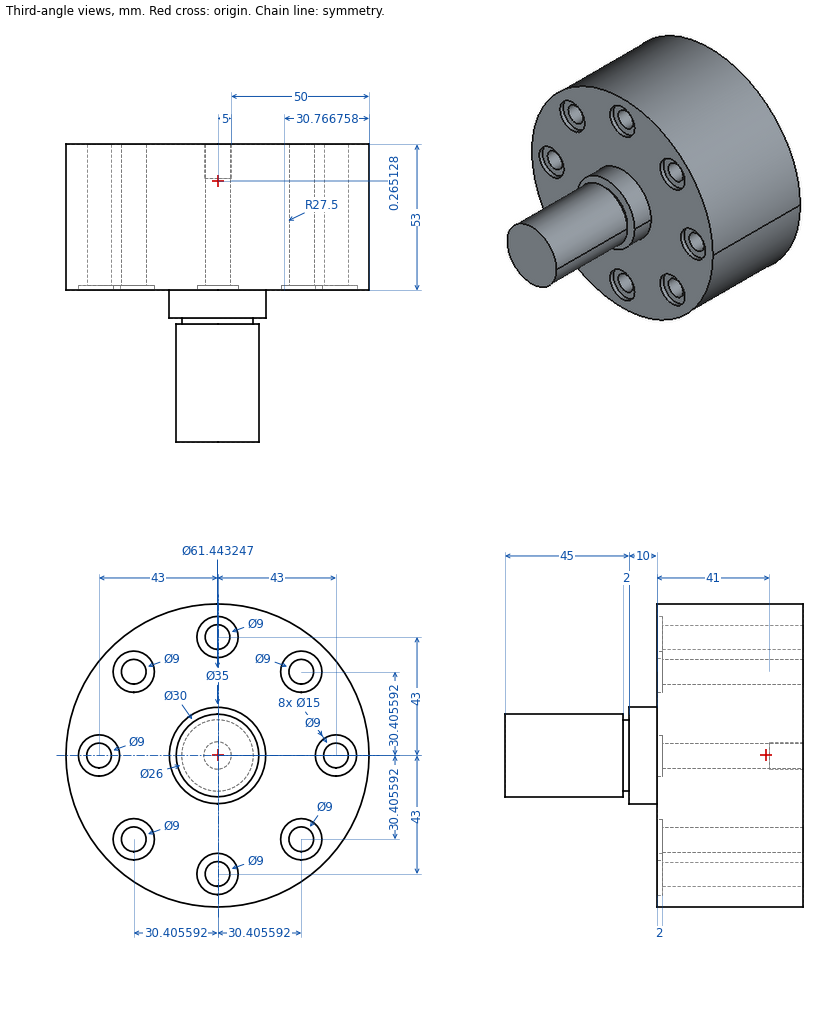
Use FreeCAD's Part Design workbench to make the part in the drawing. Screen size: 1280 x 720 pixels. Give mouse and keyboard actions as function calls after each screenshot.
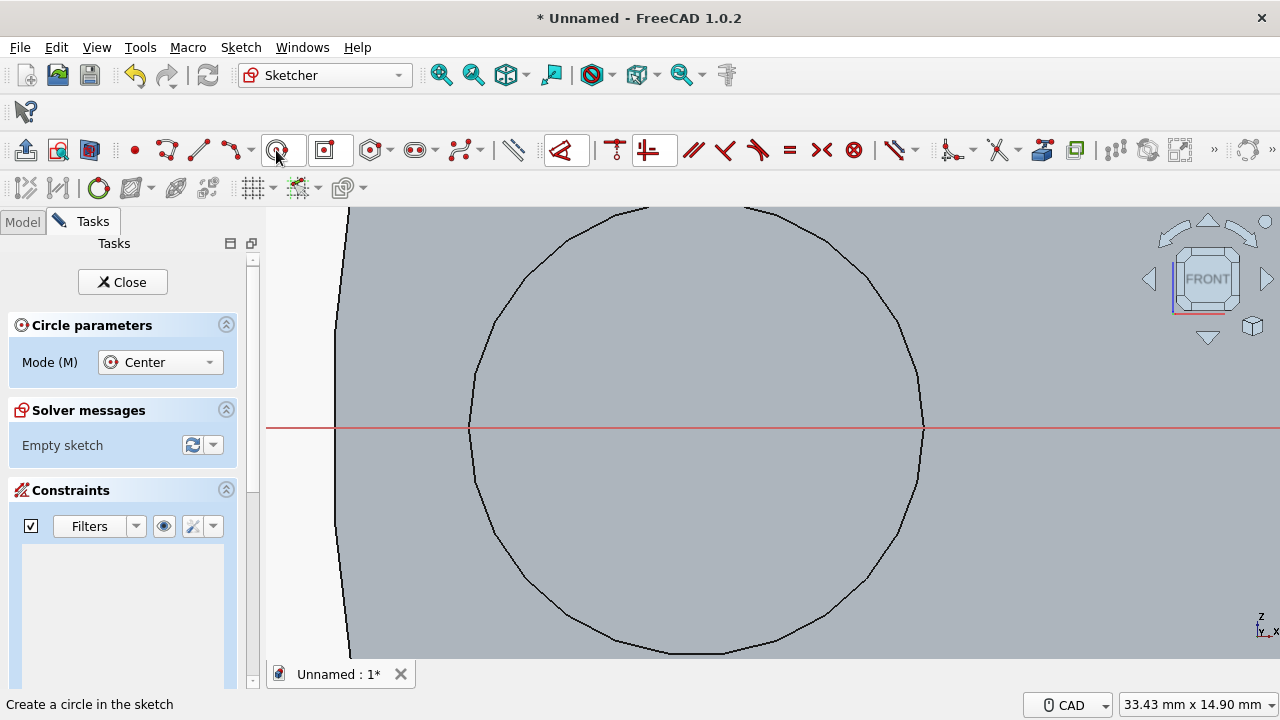
click(696, 428)
move(793, 331)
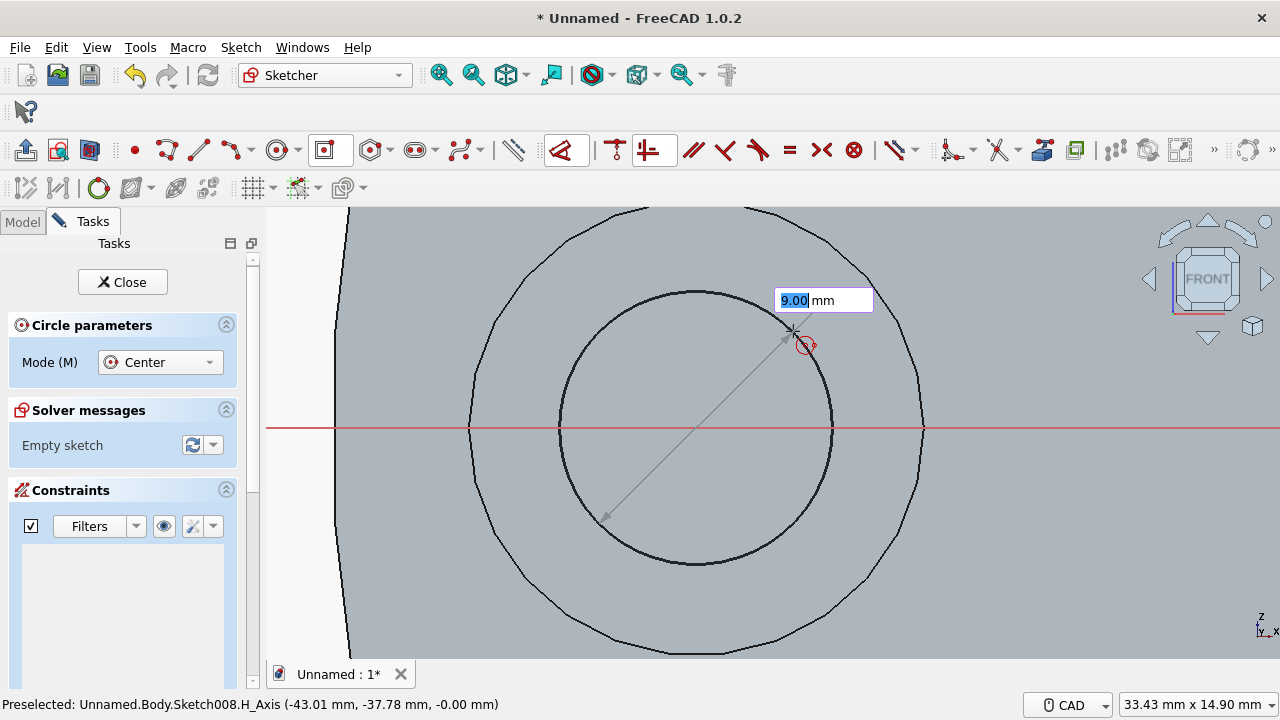
text(9)
key(Return)
key(Escape)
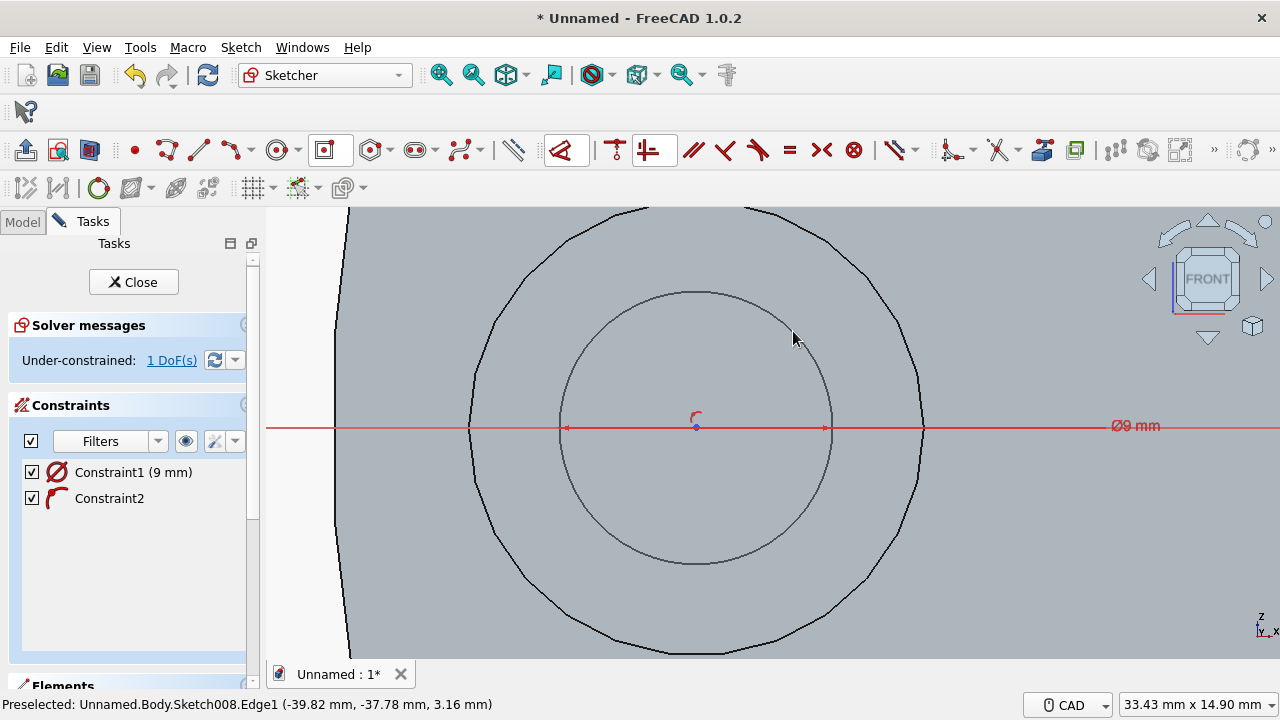
click(696, 428)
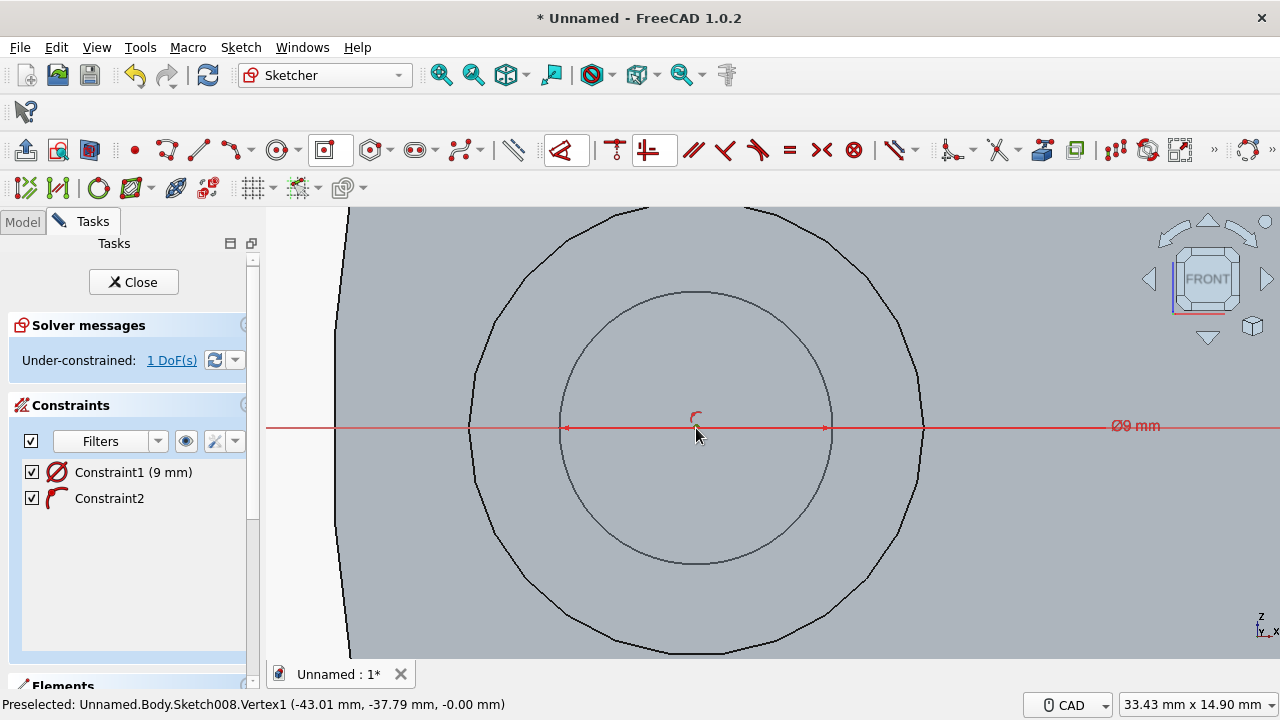
key(l)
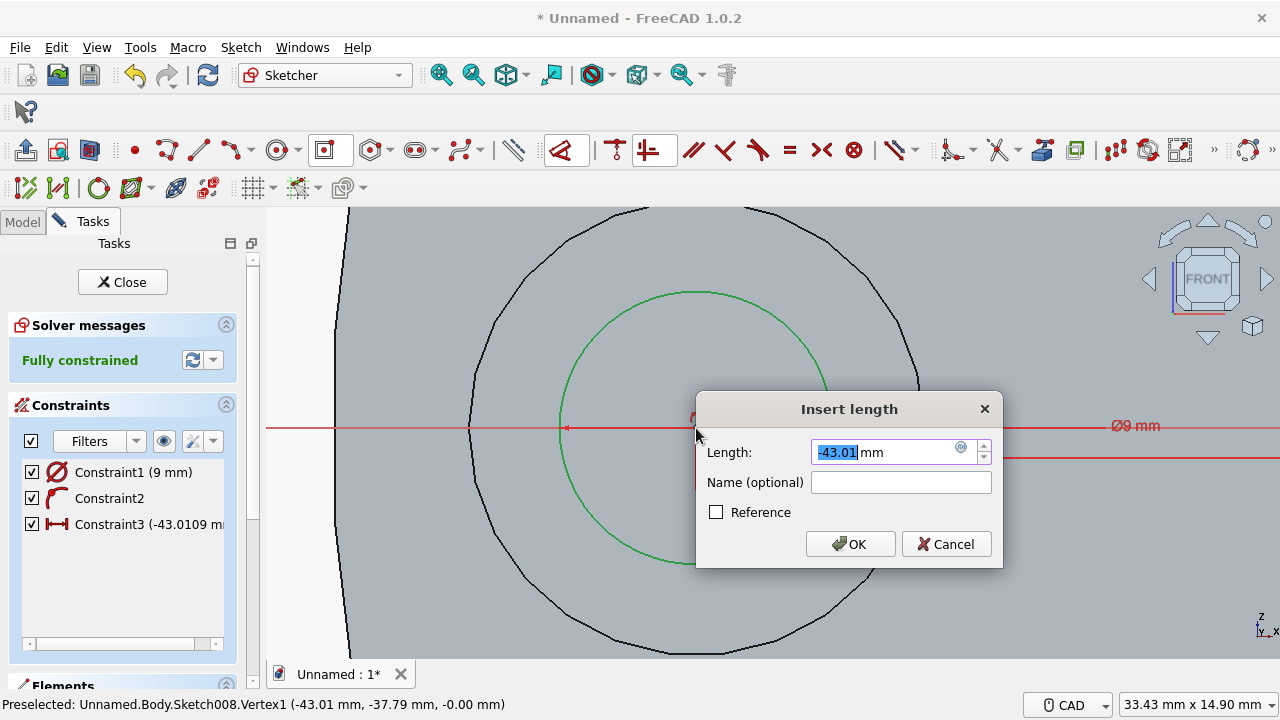
text(-43)
key(Return)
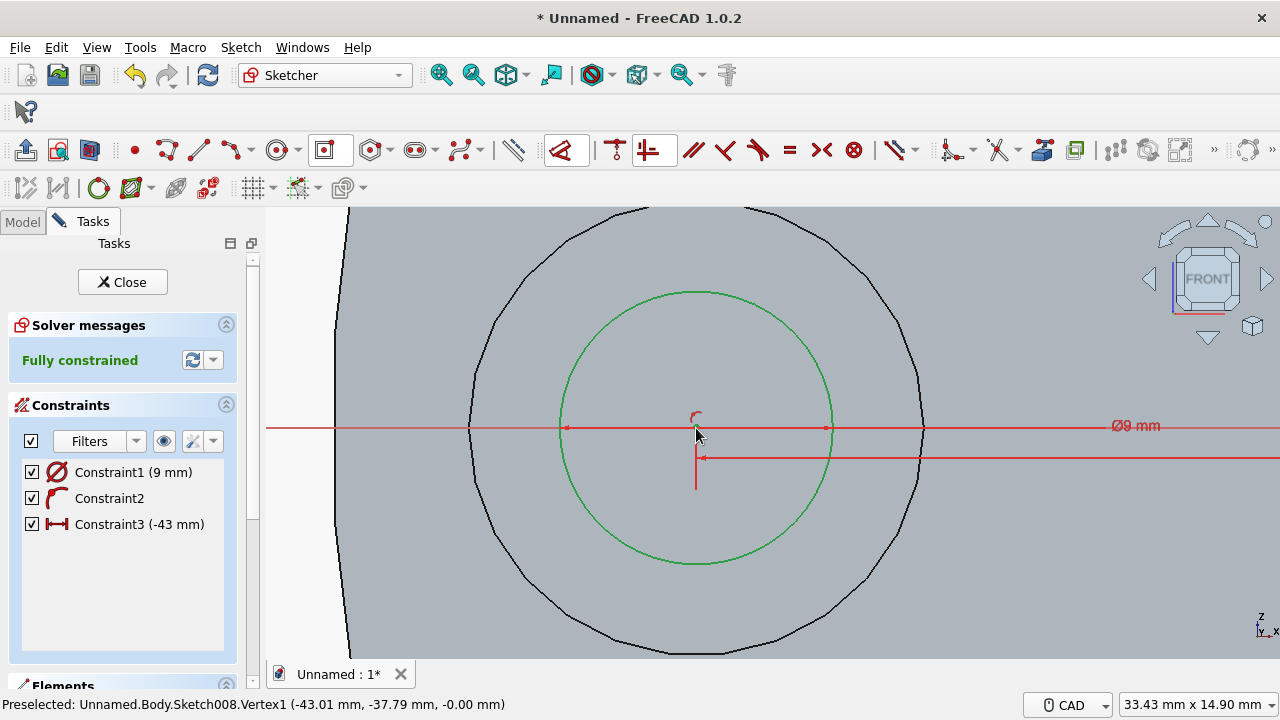
click(123, 282)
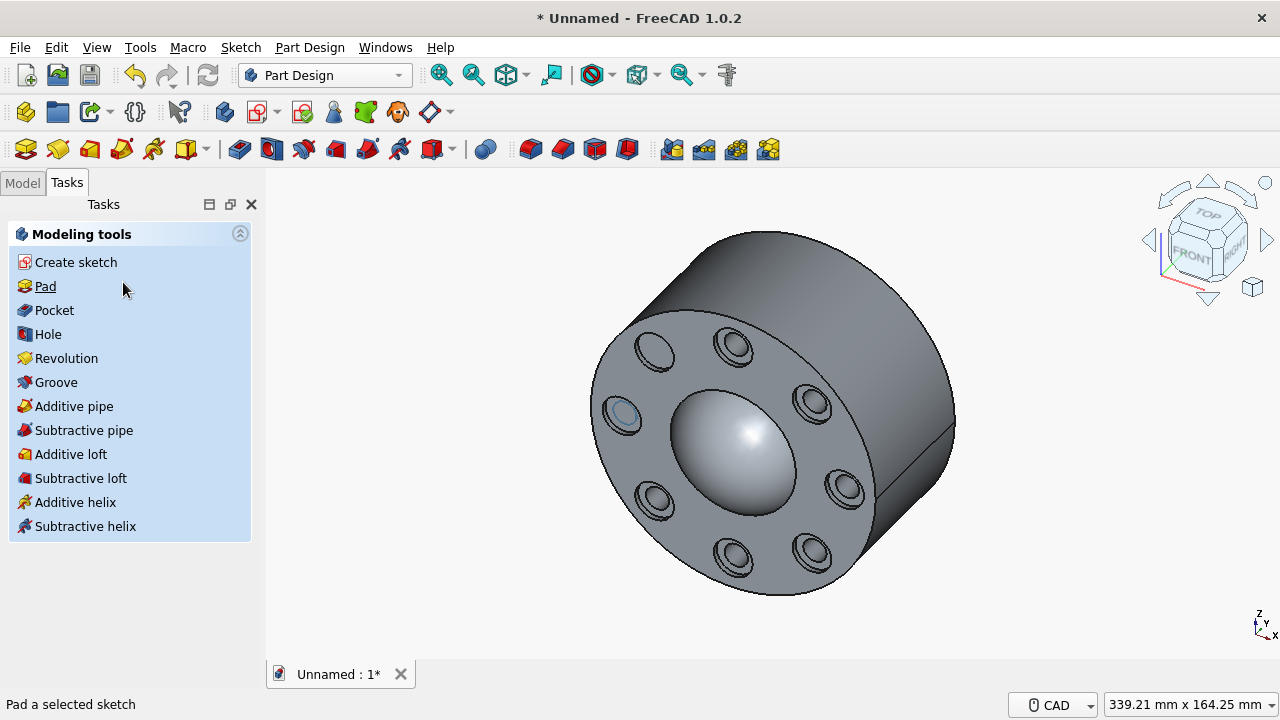
click(240, 150)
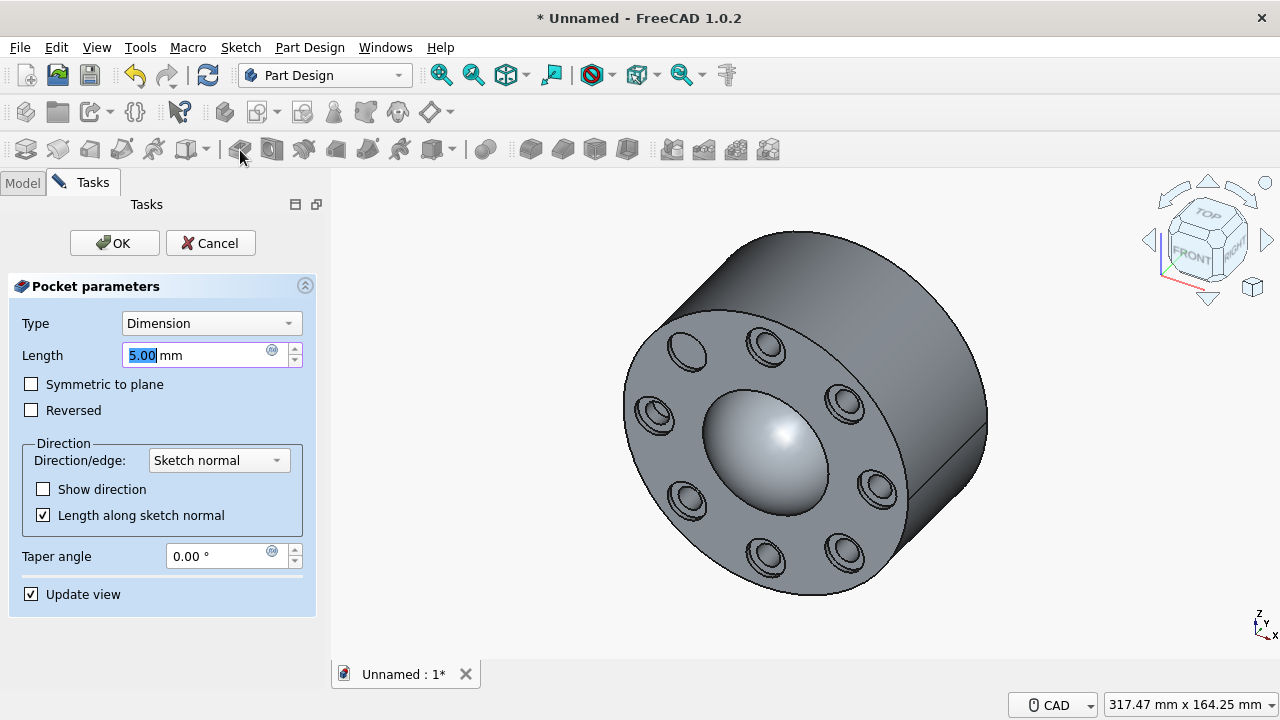
click(212, 324)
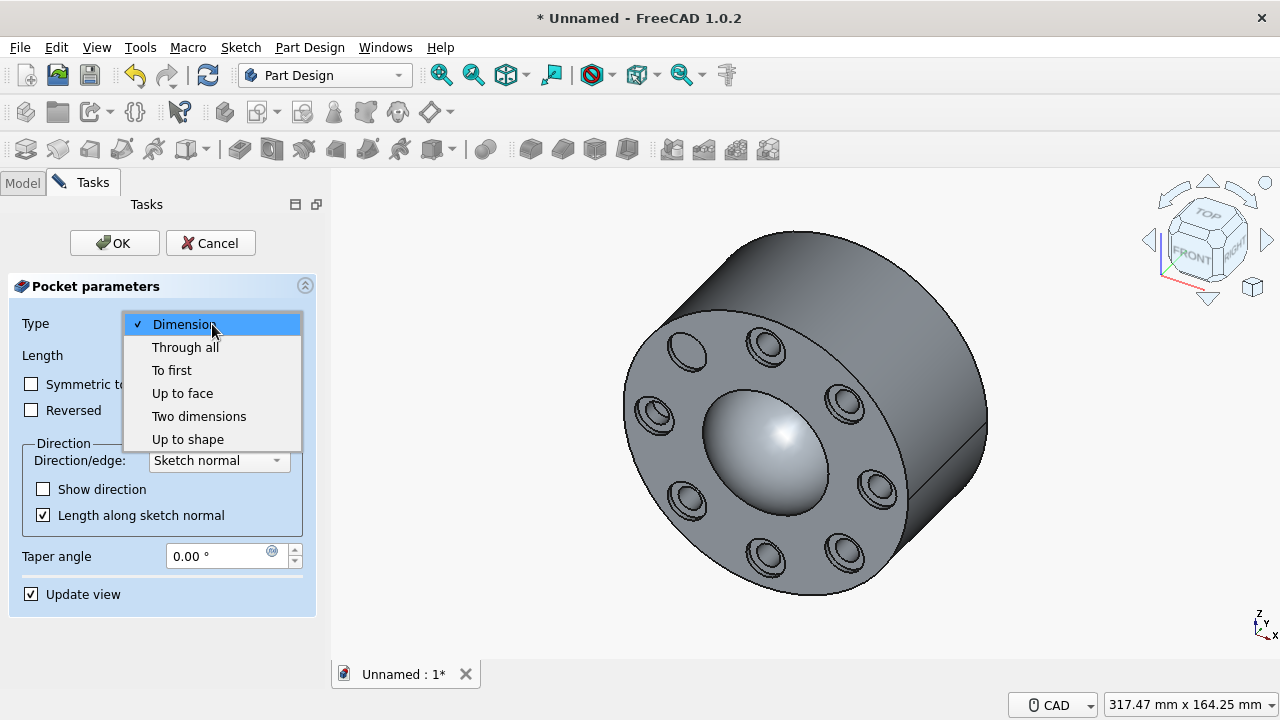
click(212, 370)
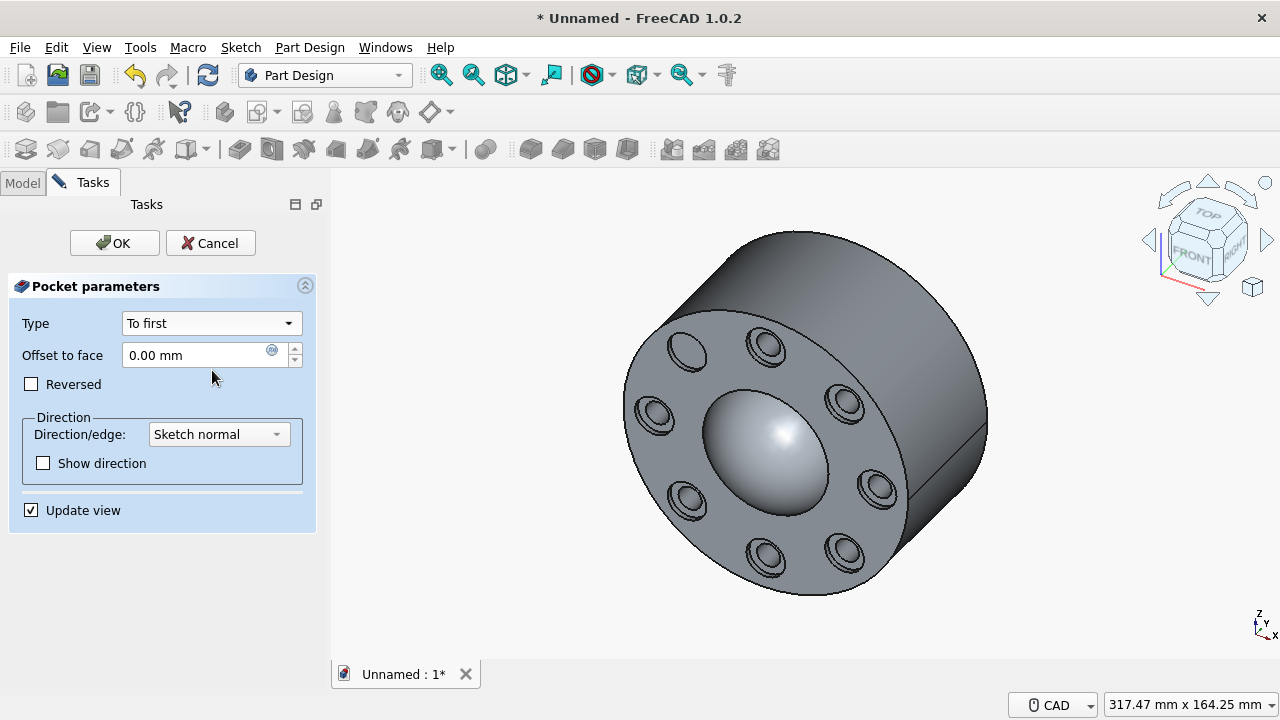
click(115, 243)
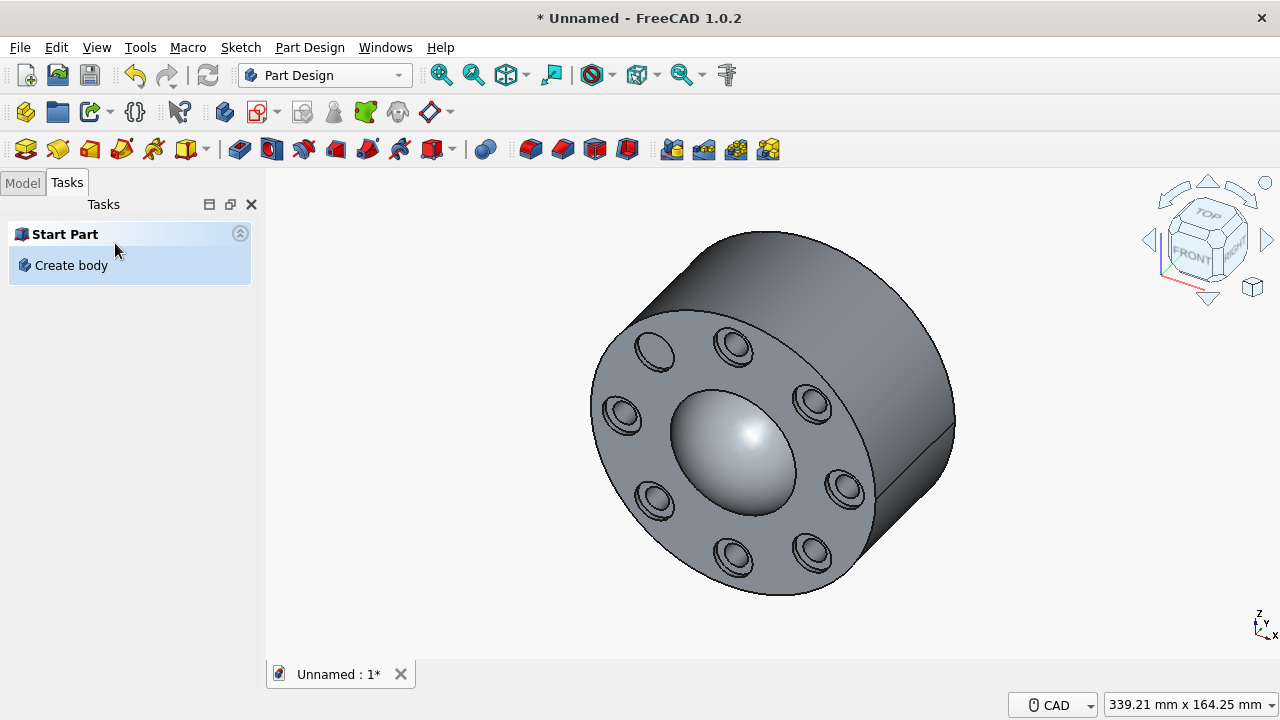
click(658, 348)